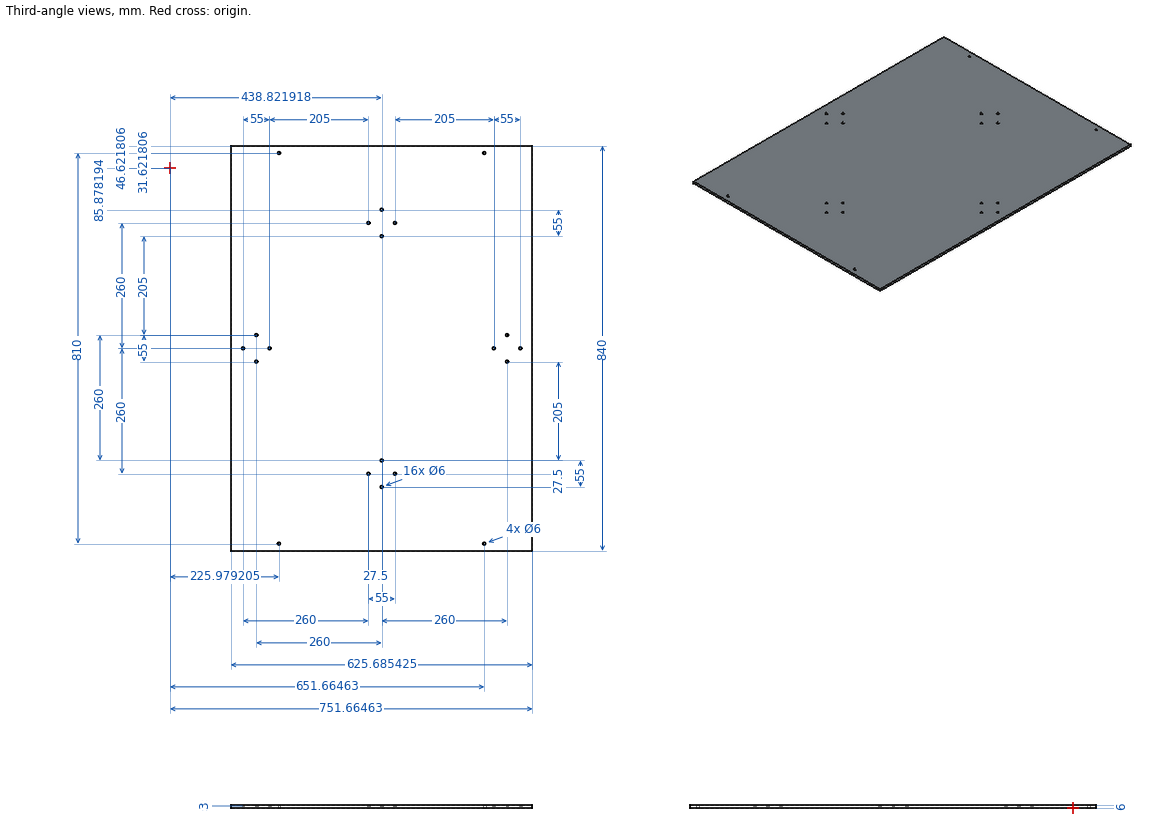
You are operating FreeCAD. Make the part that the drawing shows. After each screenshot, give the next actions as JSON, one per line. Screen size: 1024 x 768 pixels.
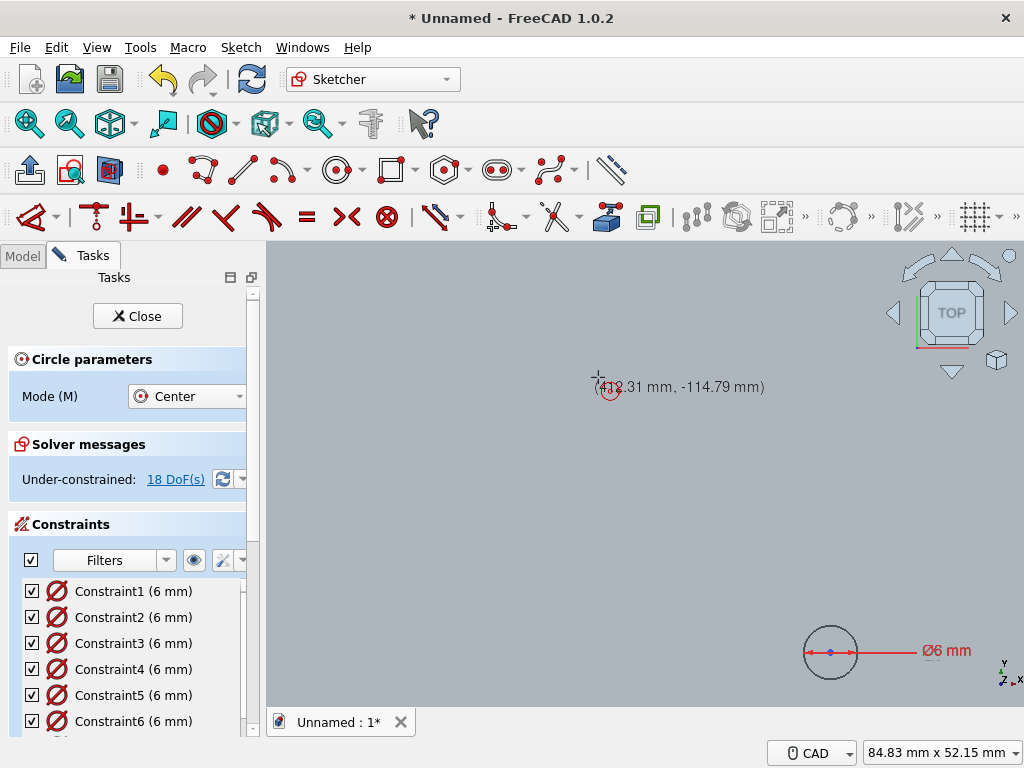
{"action": "scroll", "coordinate": [598, 377], "scroll_direction": "down", "scroll_amount": 15}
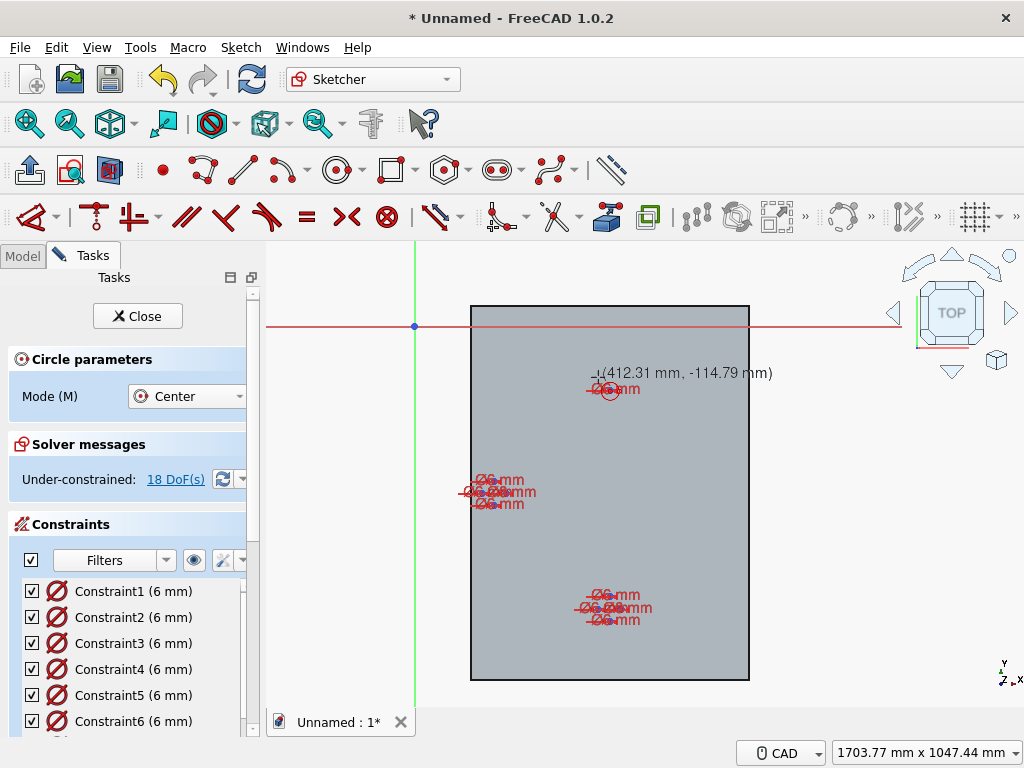
{"action": "left_click", "coordinate": [598, 377]}
{"action": "mouse_move", "coordinate": [599, 376]}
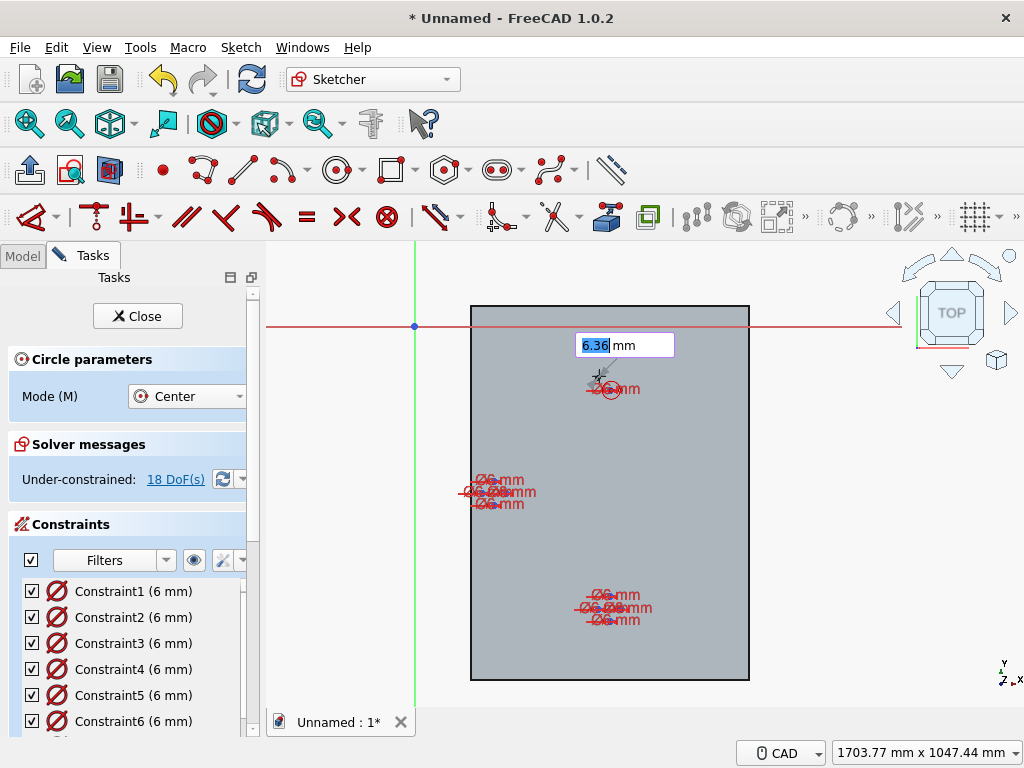
{"action": "type", "text": "6"}
{"action": "key", "text": "Return"}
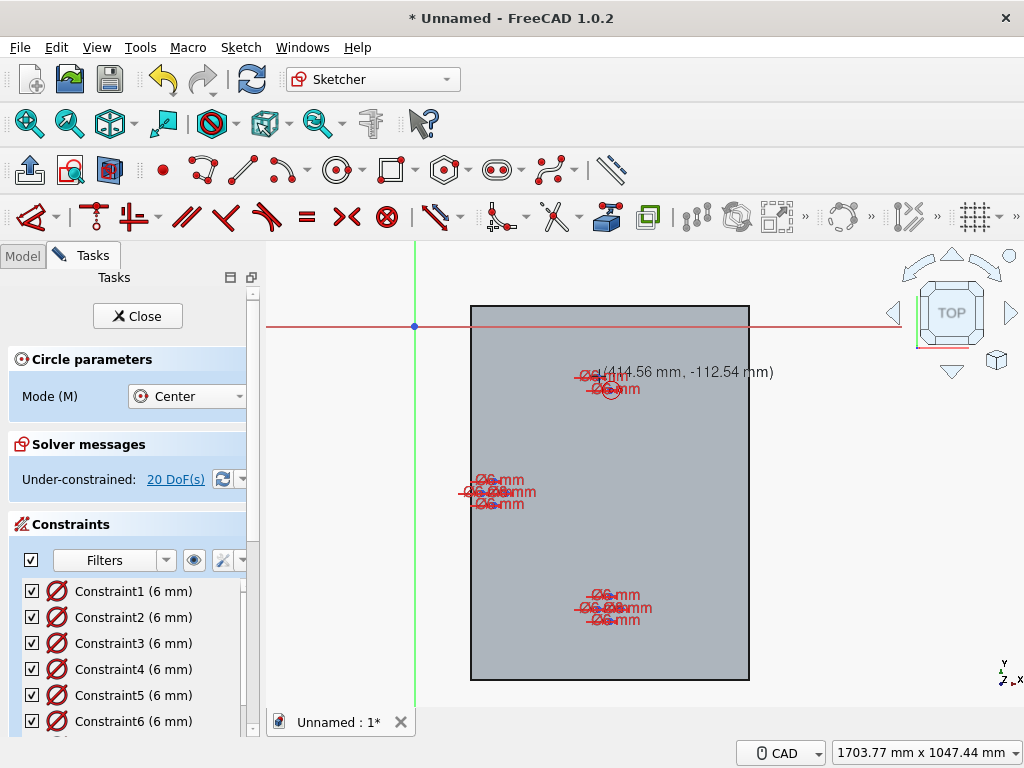
{"action": "scroll", "coordinate": [610, 365], "scroll_direction": "up", "scroll_amount": 15}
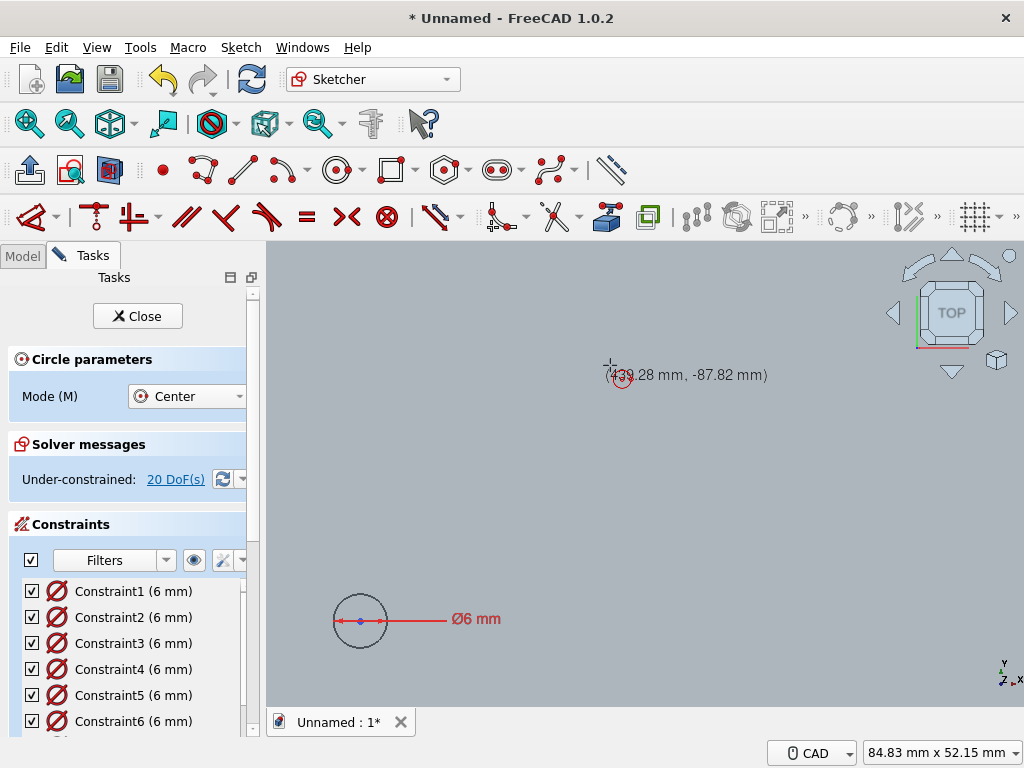
{"action": "scroll", "coordinate": [610, 365], "scroll_direction": "down", "scroll_amount": 15}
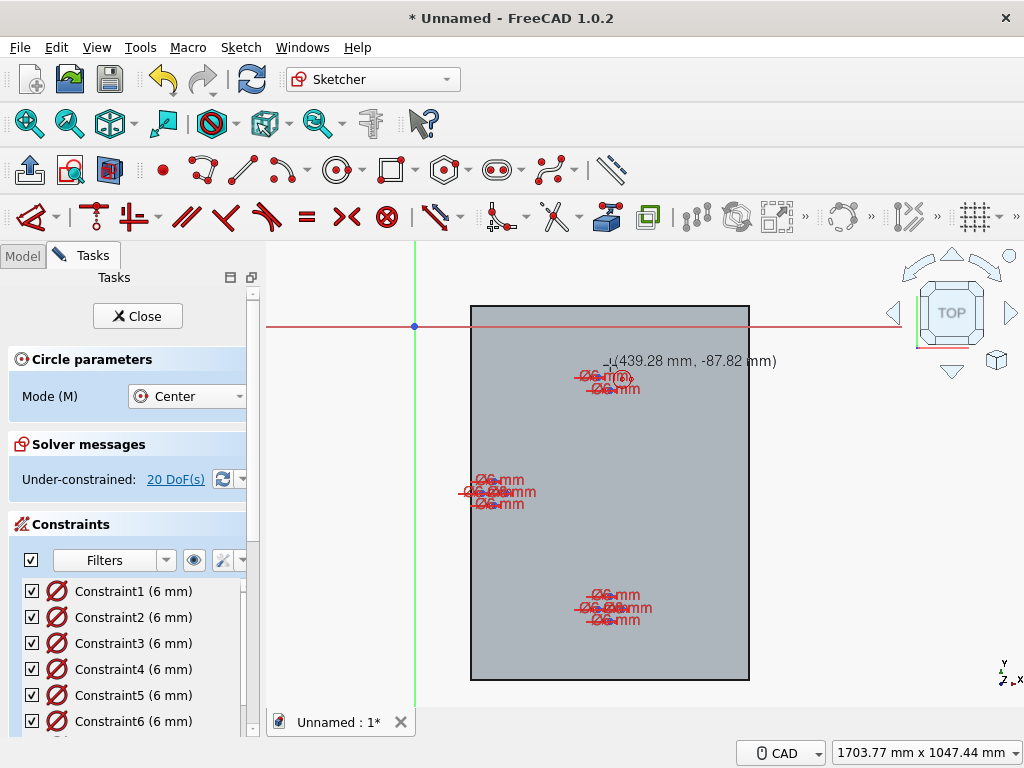
{"action": "left_click", "coordinate": [610, 365]}
{"action": "mouse_move", "coordinate": [611, 364]}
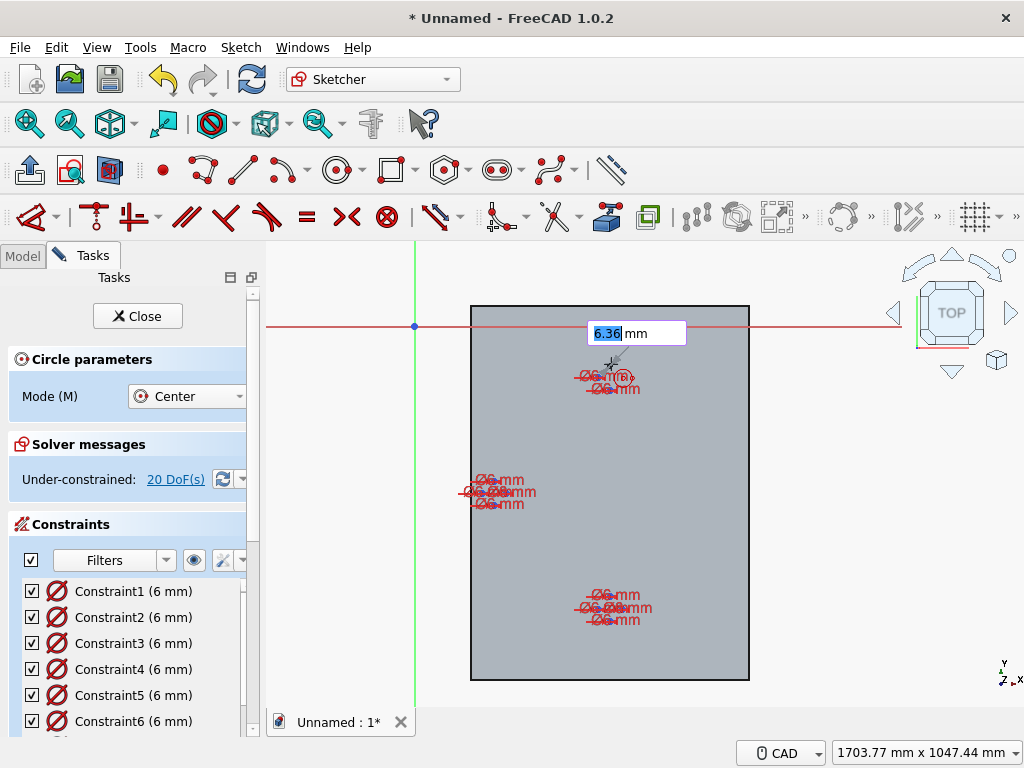
{"action": "type", "text": "6"}
{"action": "key", "text": "Return"}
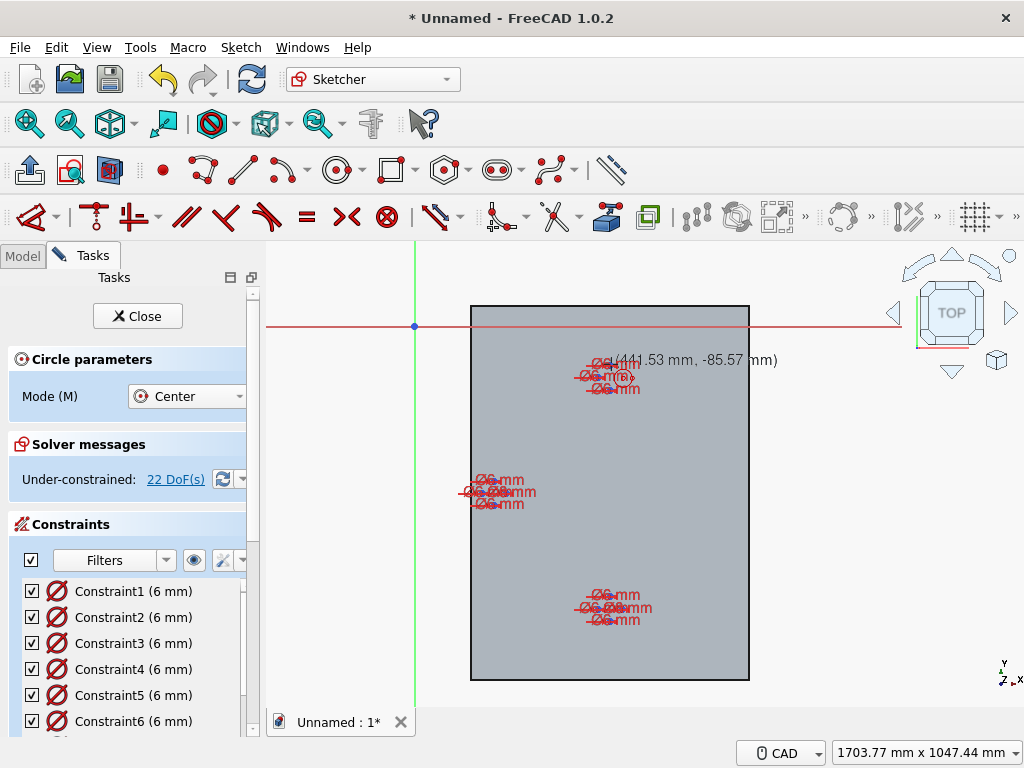
{"action": "scroll", "coordinate": [622, 377], "scroll_direction": "up", "scroll_amount": 15}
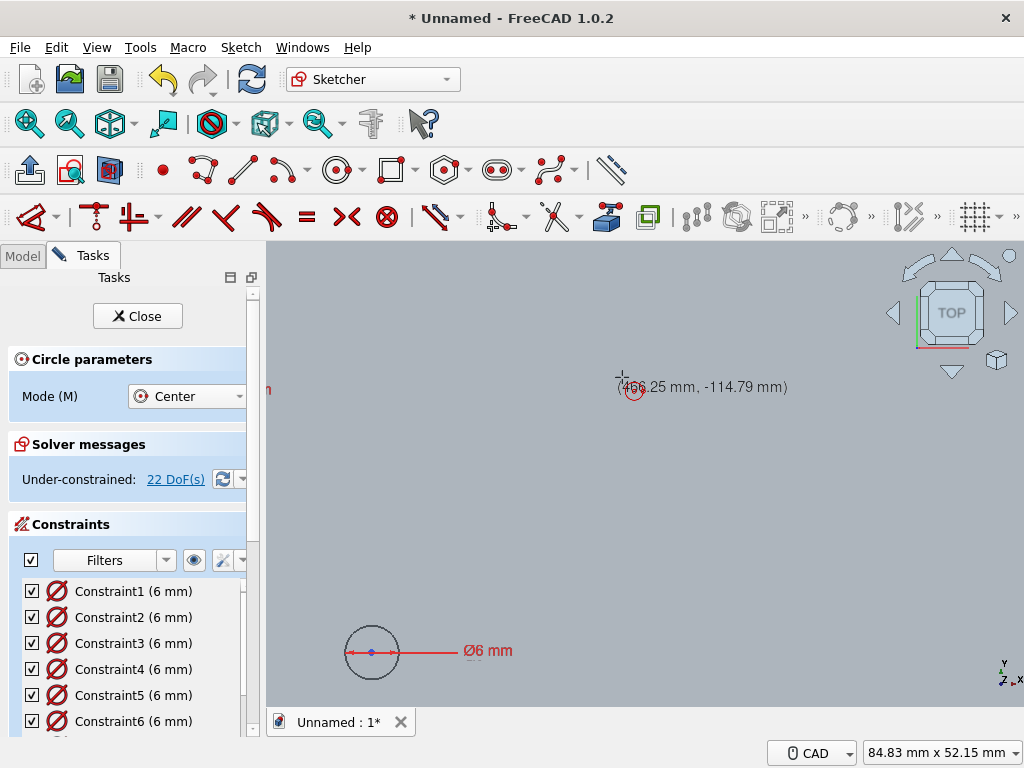
{"action": "scroll", "coordinate": [622, 377], "scroll_direction": "down", "scroll_amount": 15}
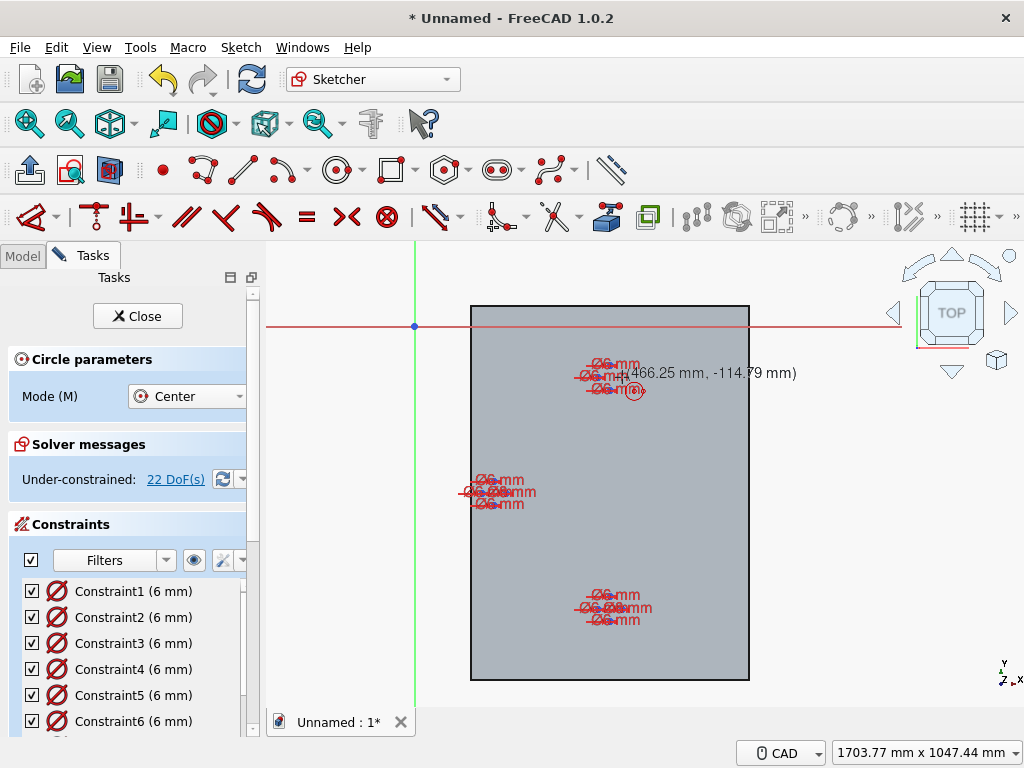
{"action": "left_click", "coordinate": [622, 377]}
{"action": "mouse_move", "coordinate": [623, 376]}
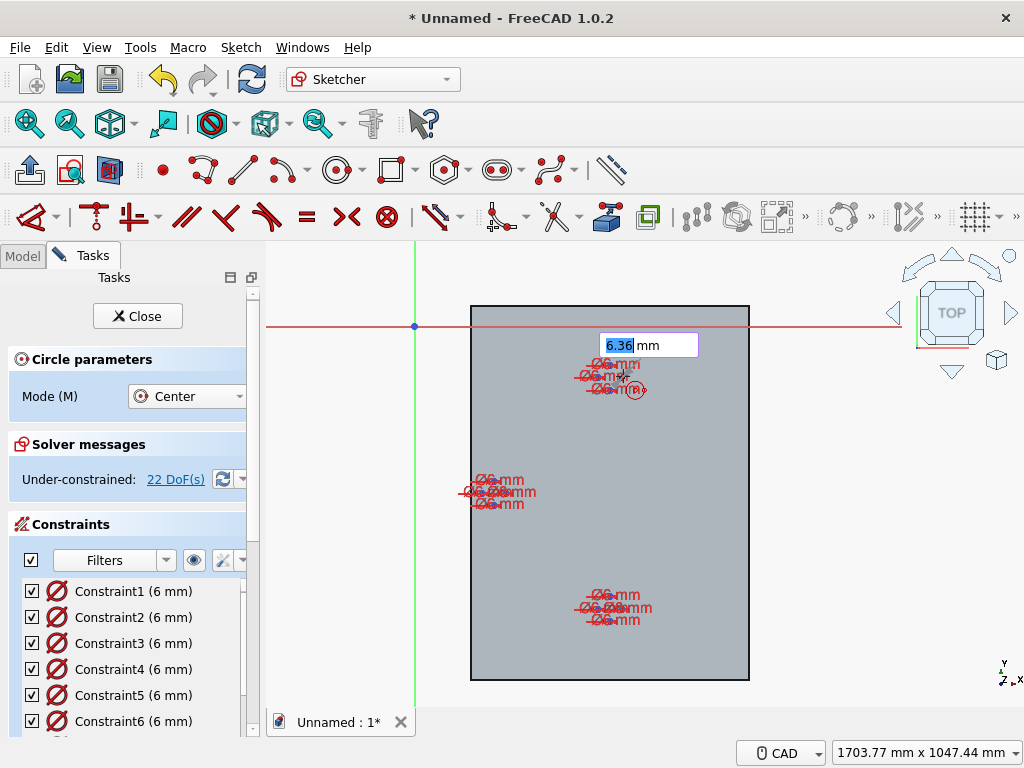
{"action": "type", "text": "6"}
{"action": "key", "text": "Return"}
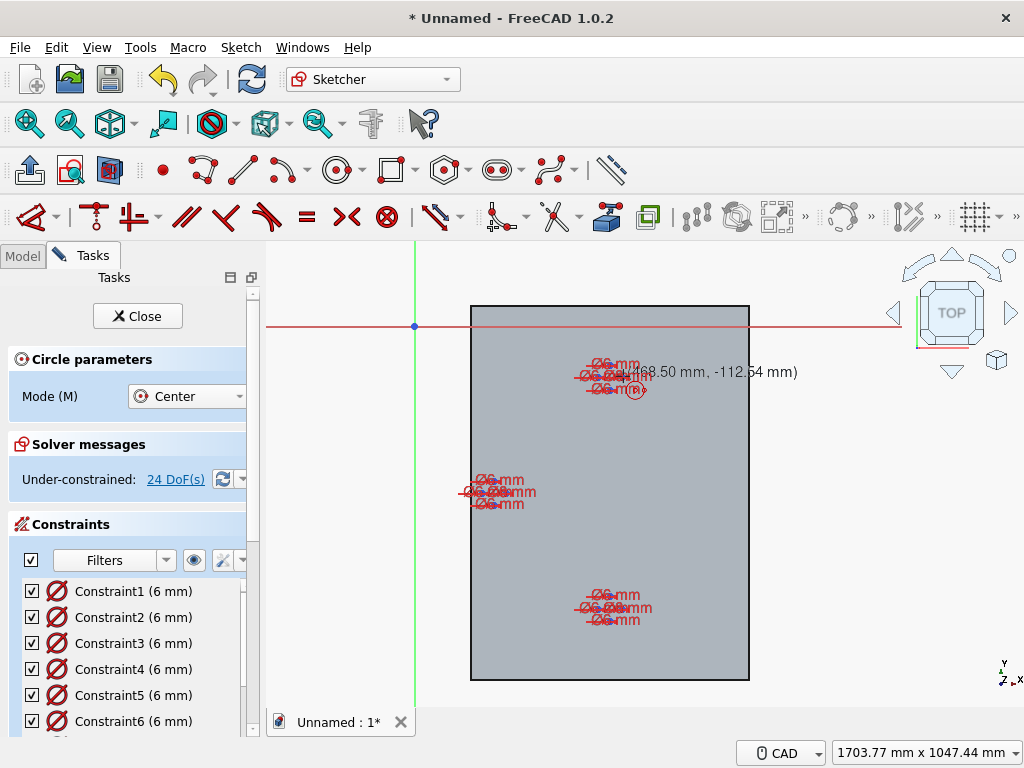
{"action": "scroll", "coordinate": [725, 505], "scroll_direction": "up", "scroll_amount": 15}